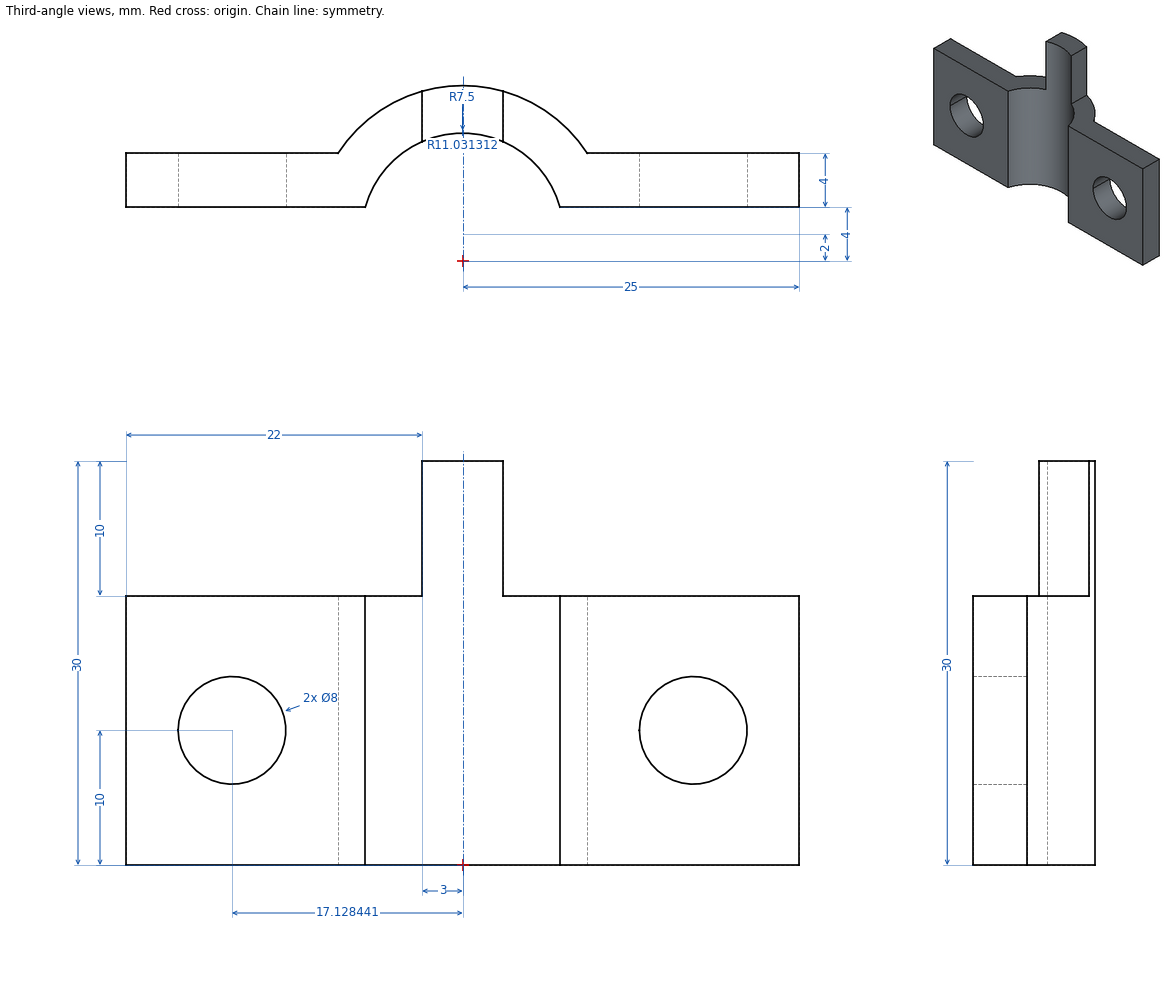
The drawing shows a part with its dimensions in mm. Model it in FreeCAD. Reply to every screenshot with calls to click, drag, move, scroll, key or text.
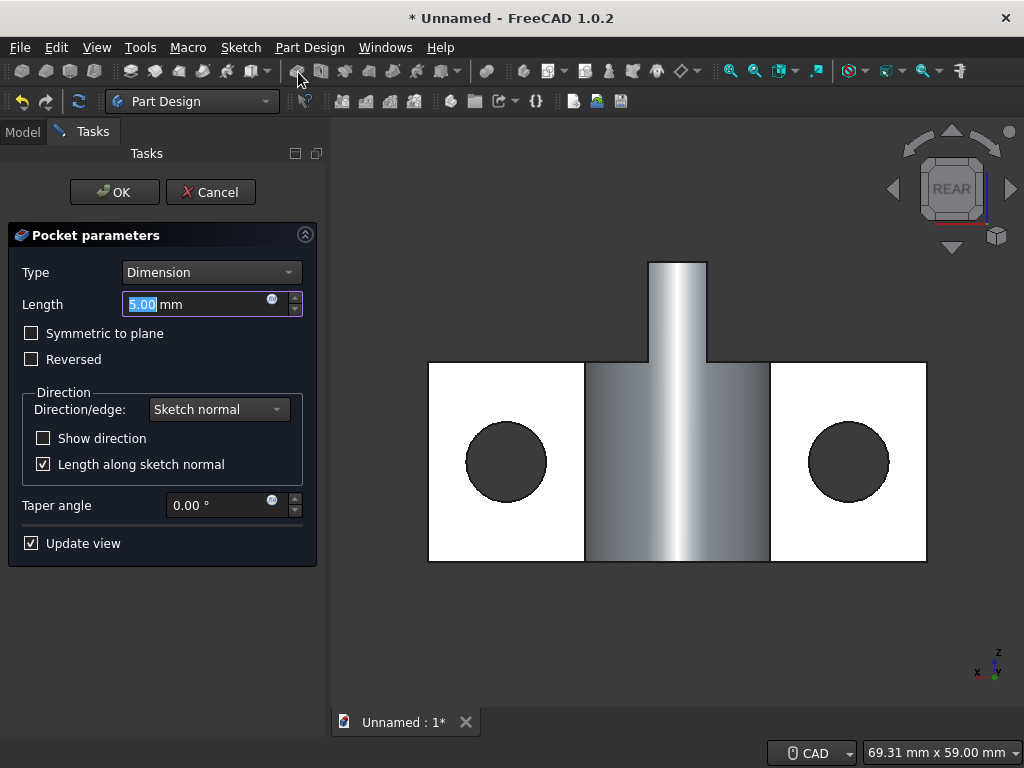
click(212, 272)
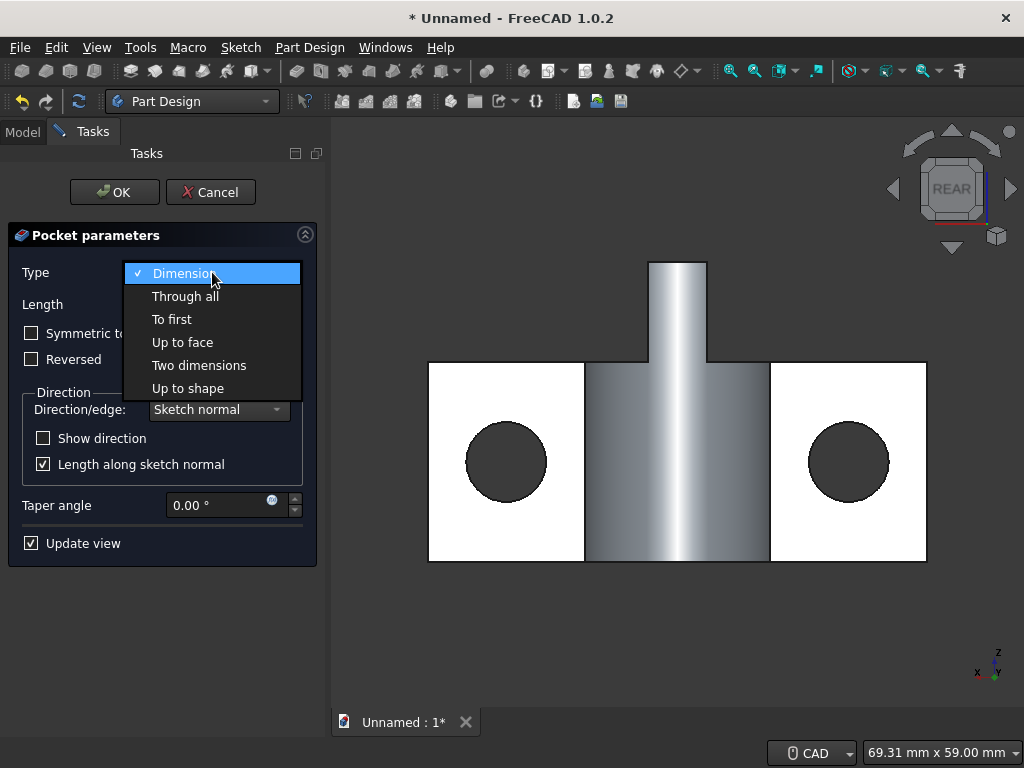
click(212, 296)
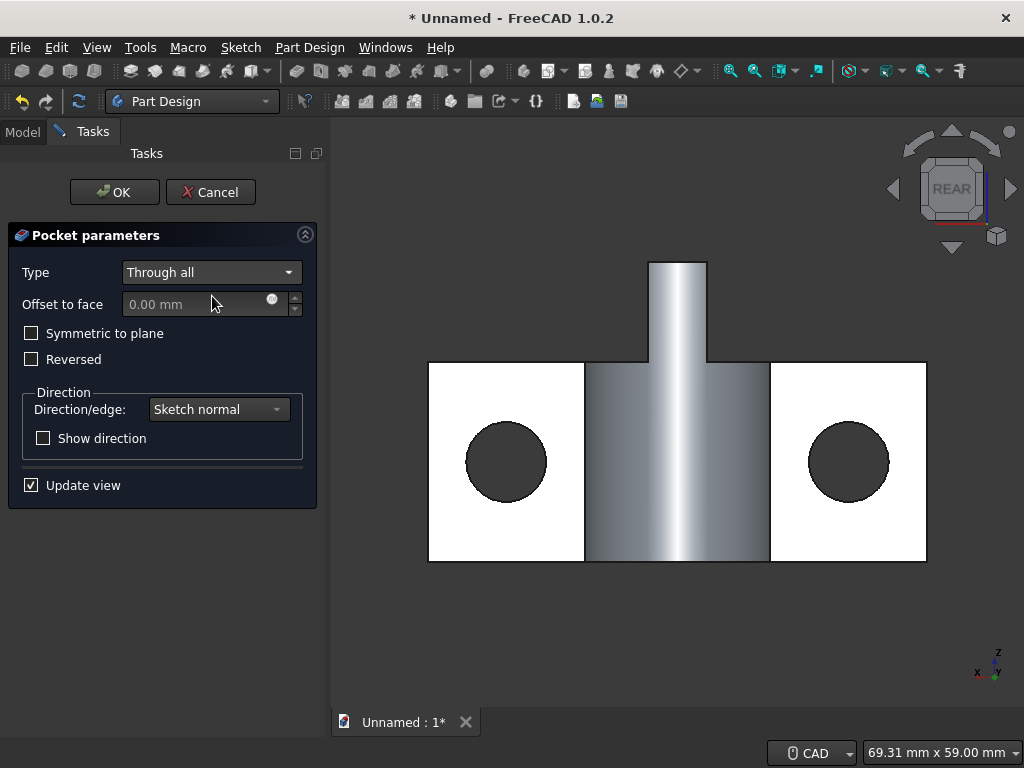
click(115, 192)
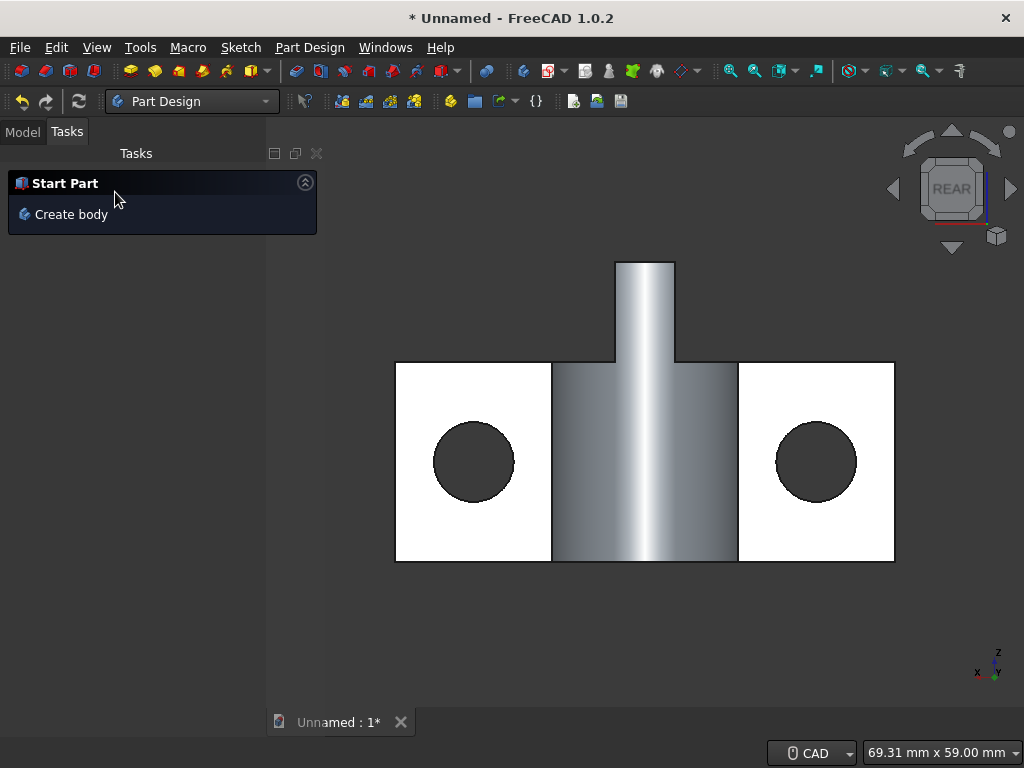
key(0)